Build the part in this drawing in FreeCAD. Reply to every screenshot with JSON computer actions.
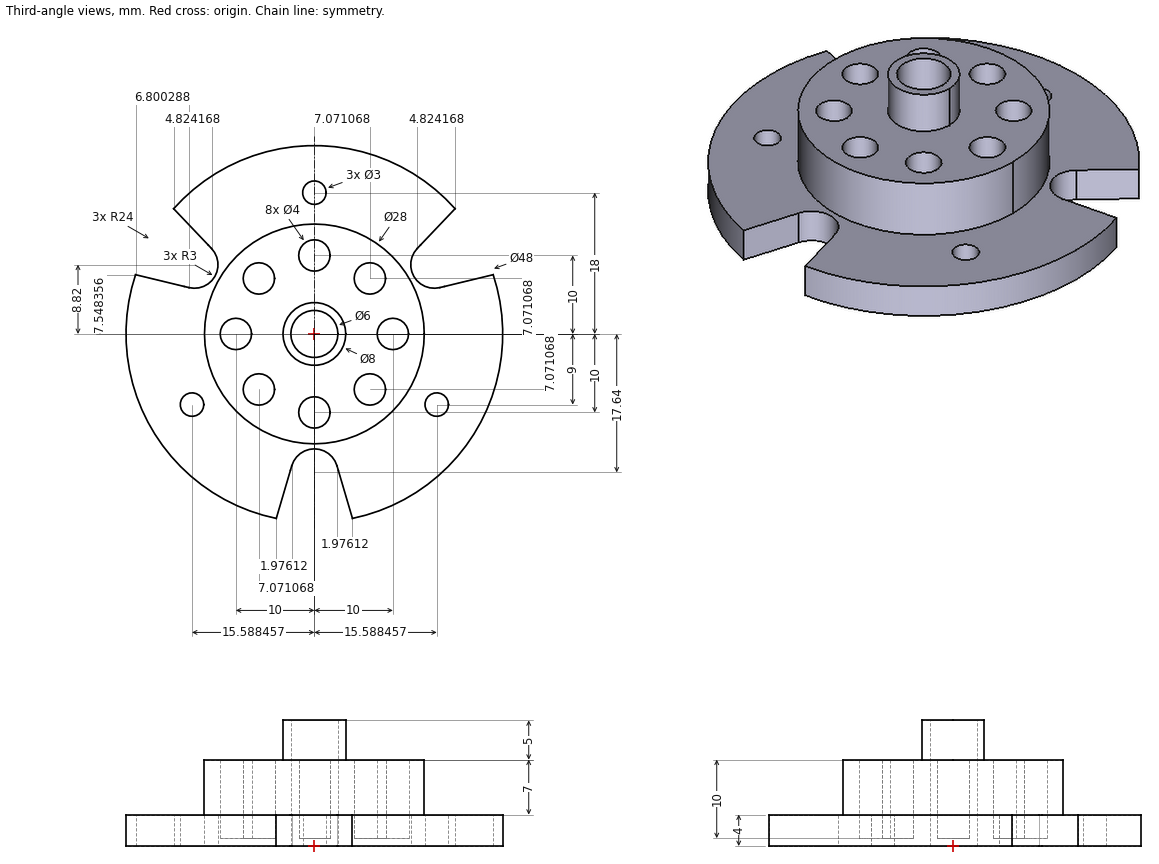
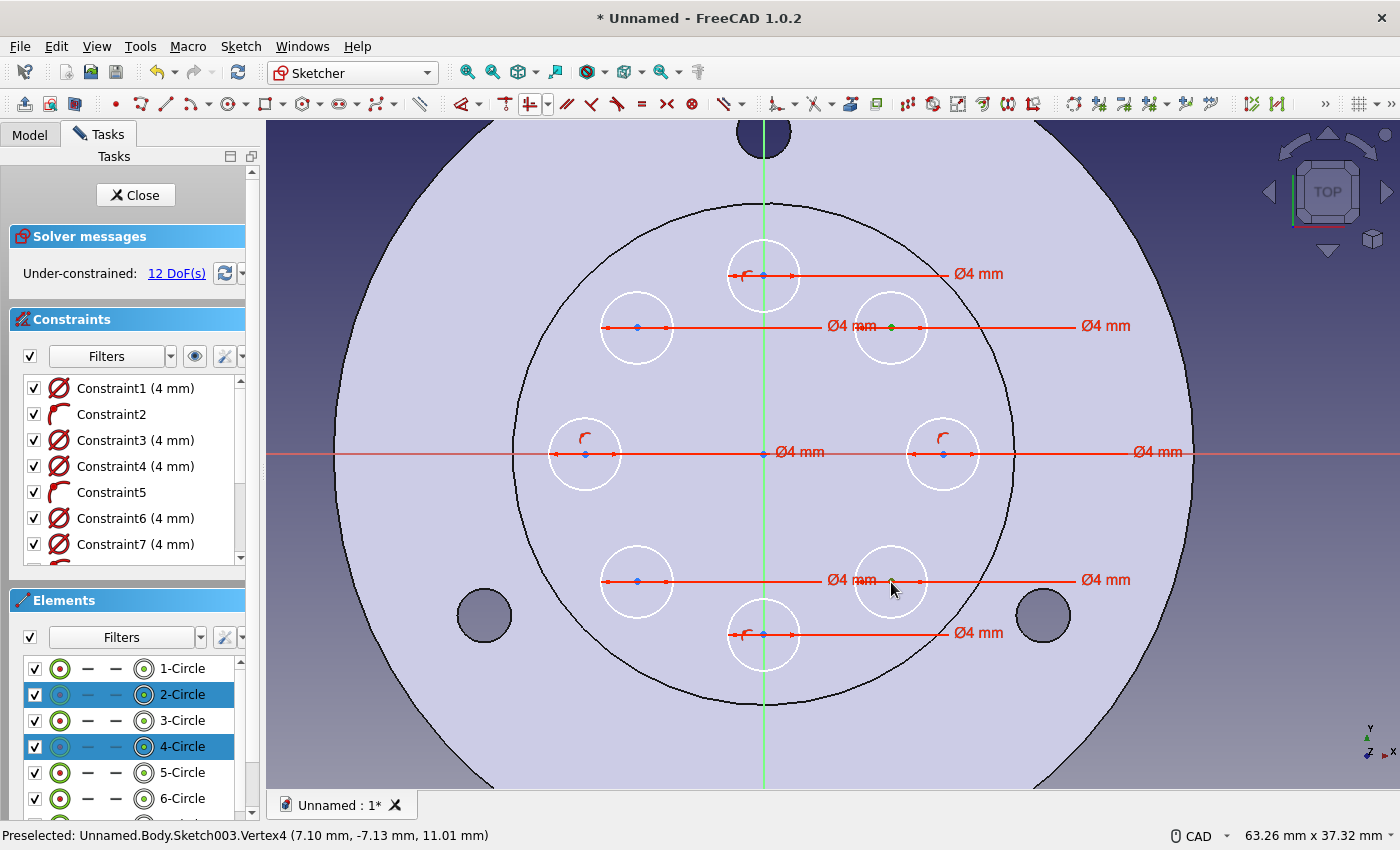
{"action": "key", "text": "v"}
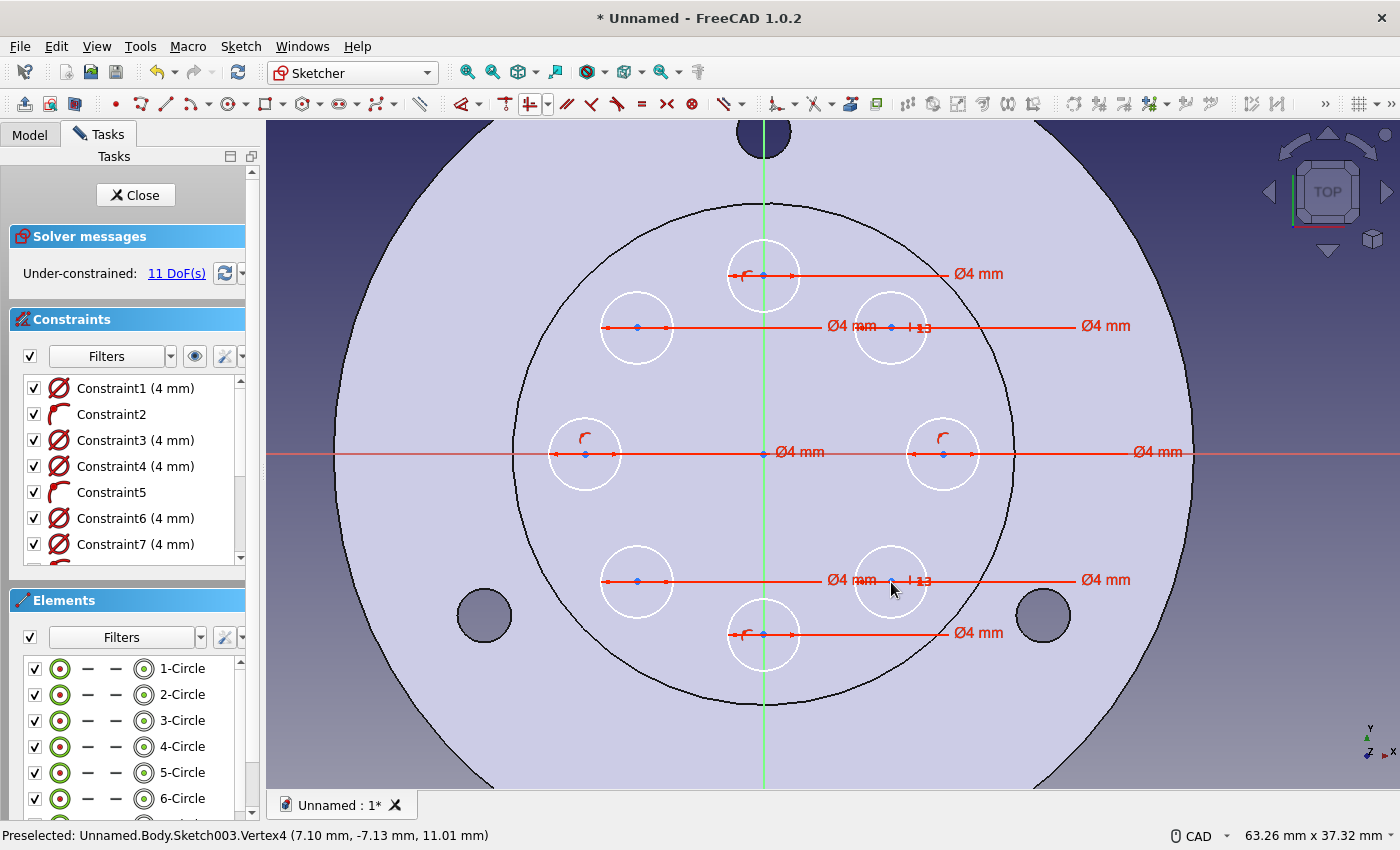
{"action": "left_click", "coordinate": [891, 582]}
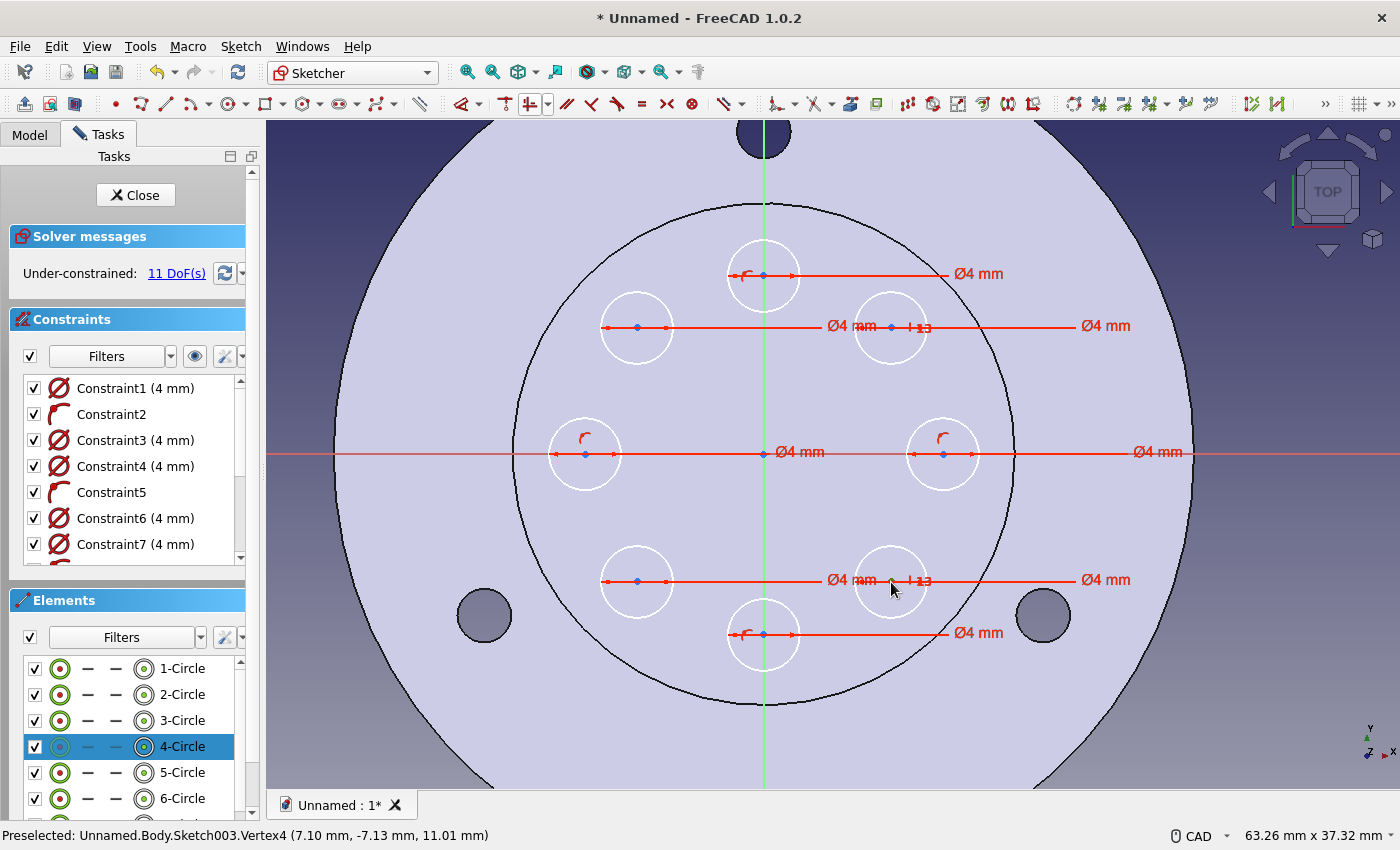
{"action": "left_click", "coordinate": [637, 582]}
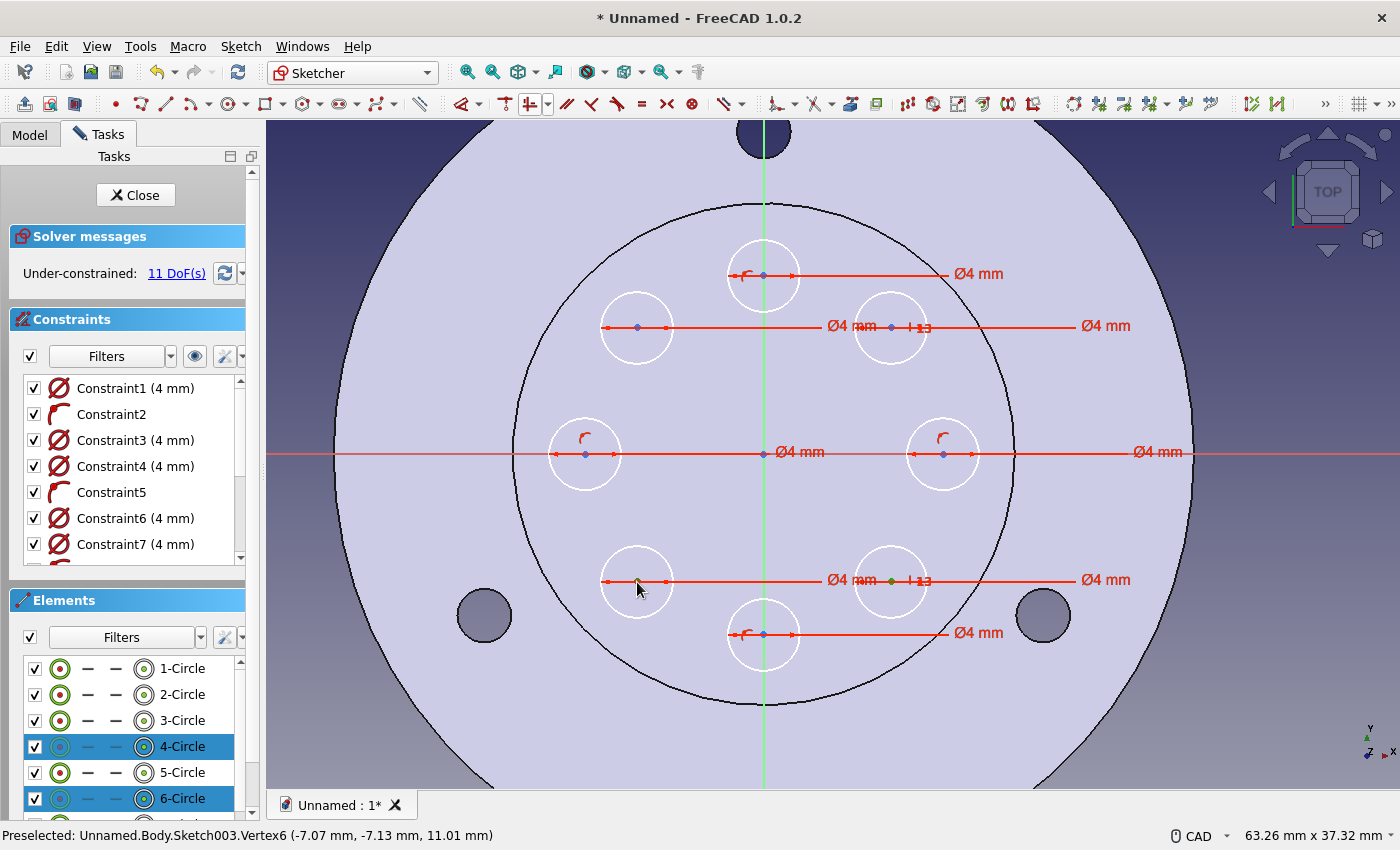
{"action": "key", "text": "h"}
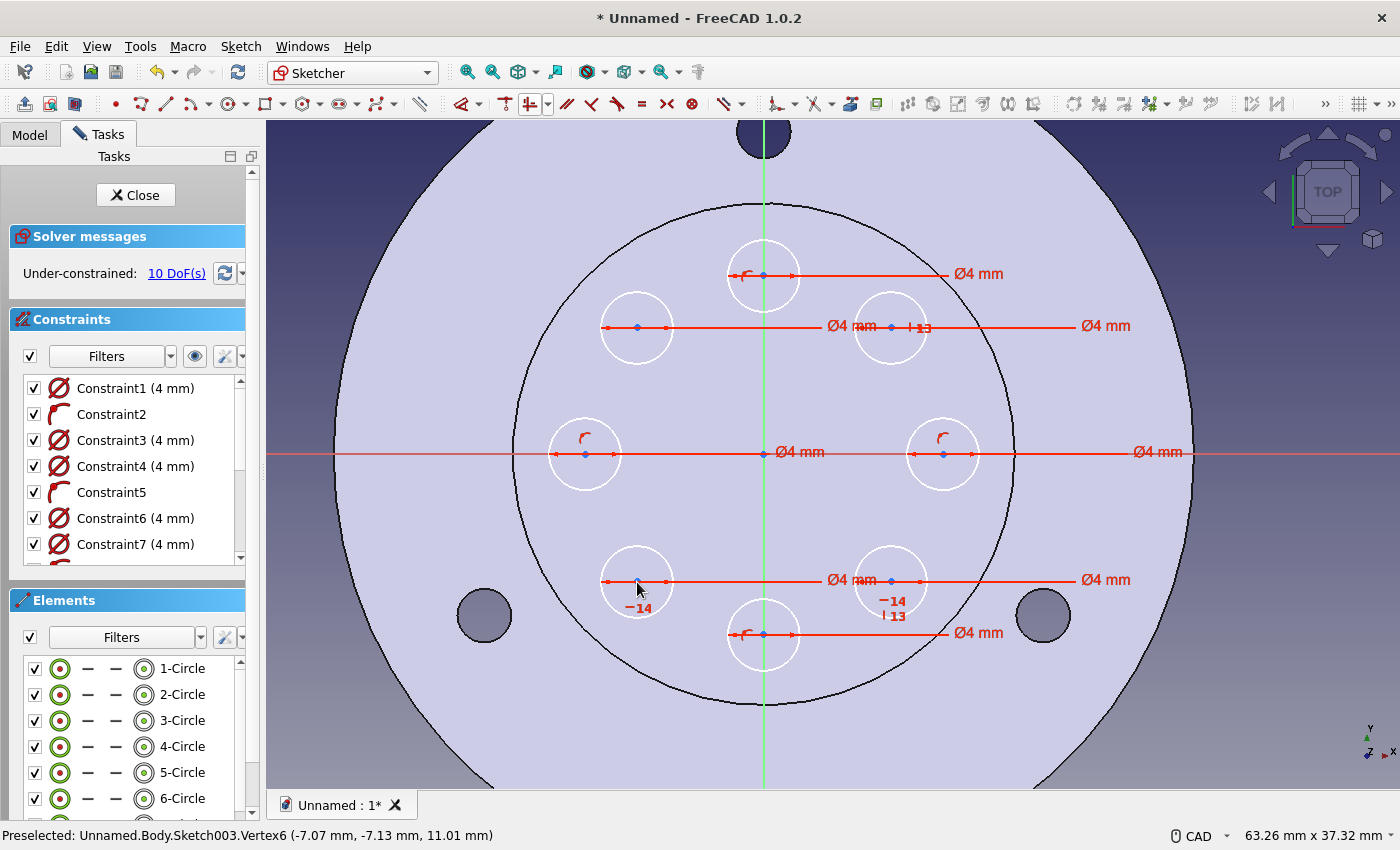
{"action": "left_click", "coordinate": [637, 582]}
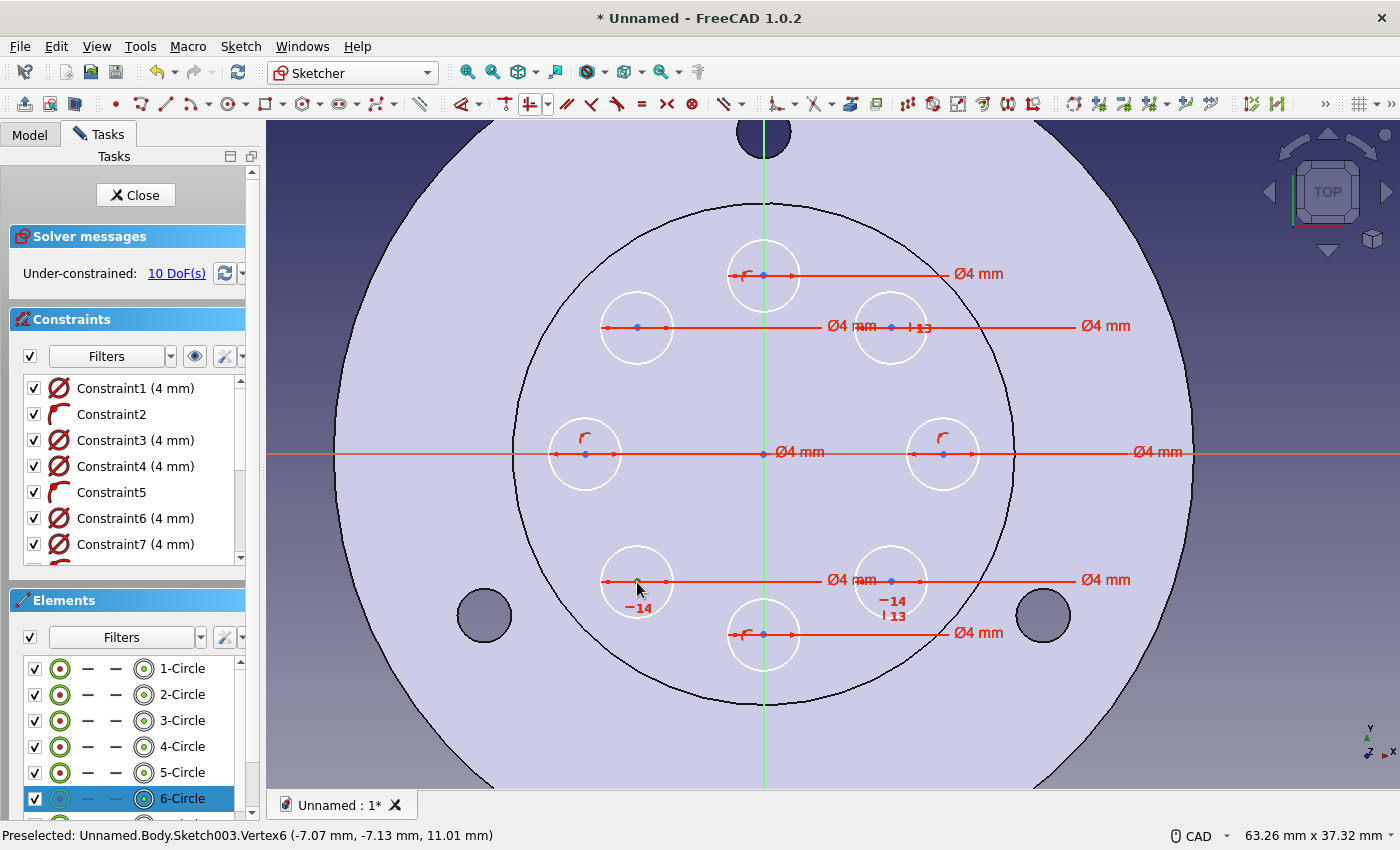
{"action": "left_click", "coordinate": [637, 328]}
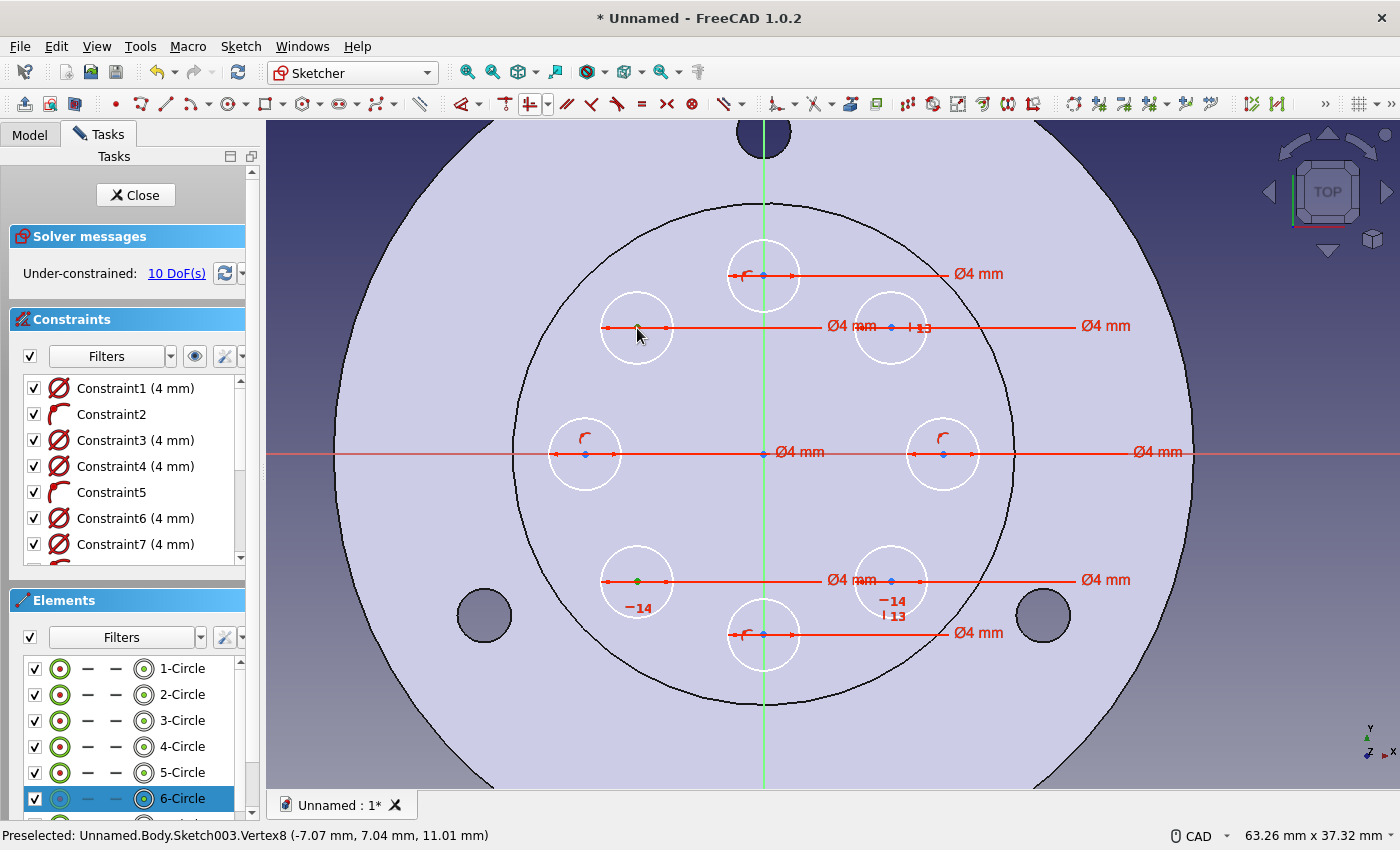
{"action": "key", "text": "v"}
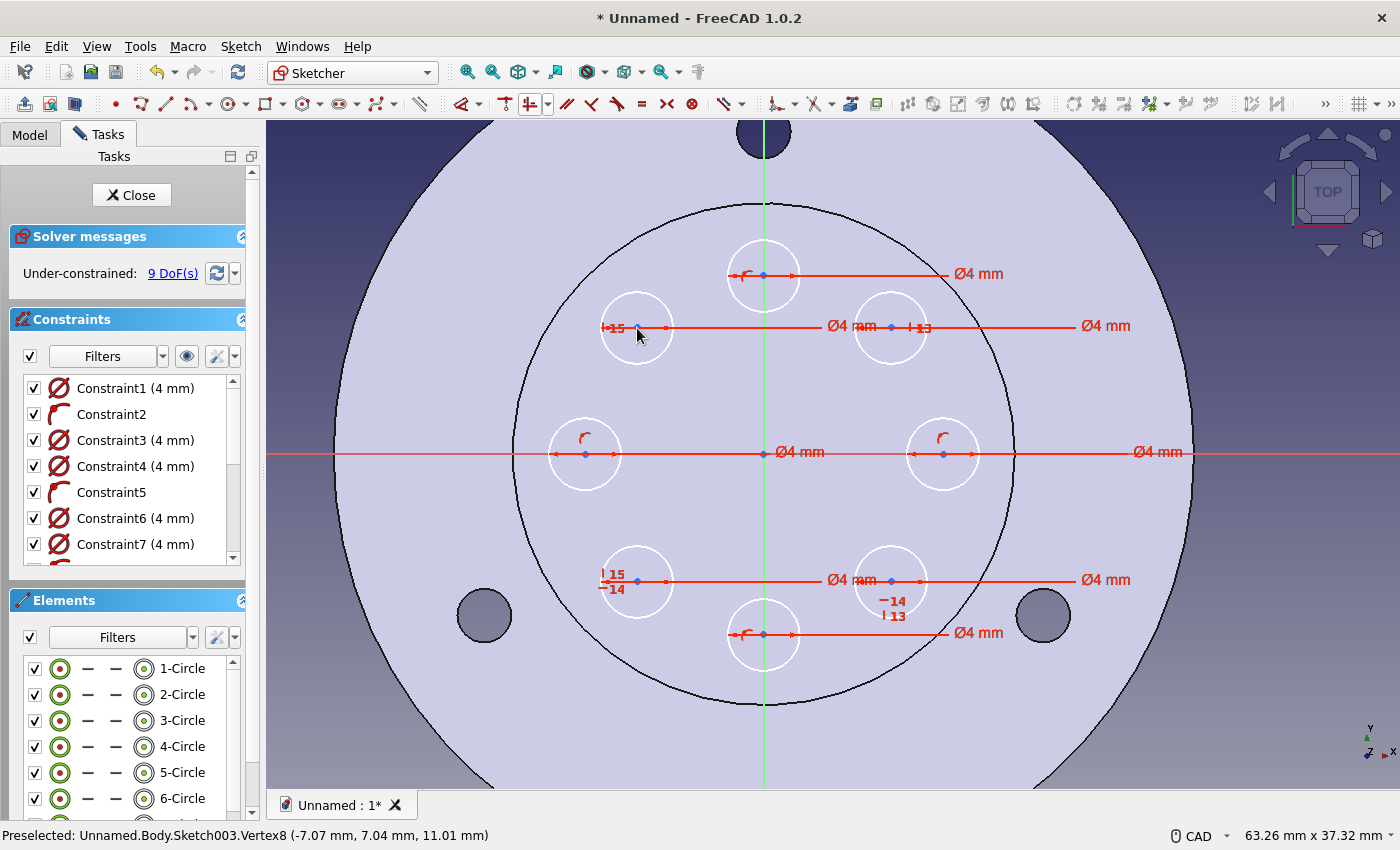
{"action": "left_click", "coordinate": [891, 328]}